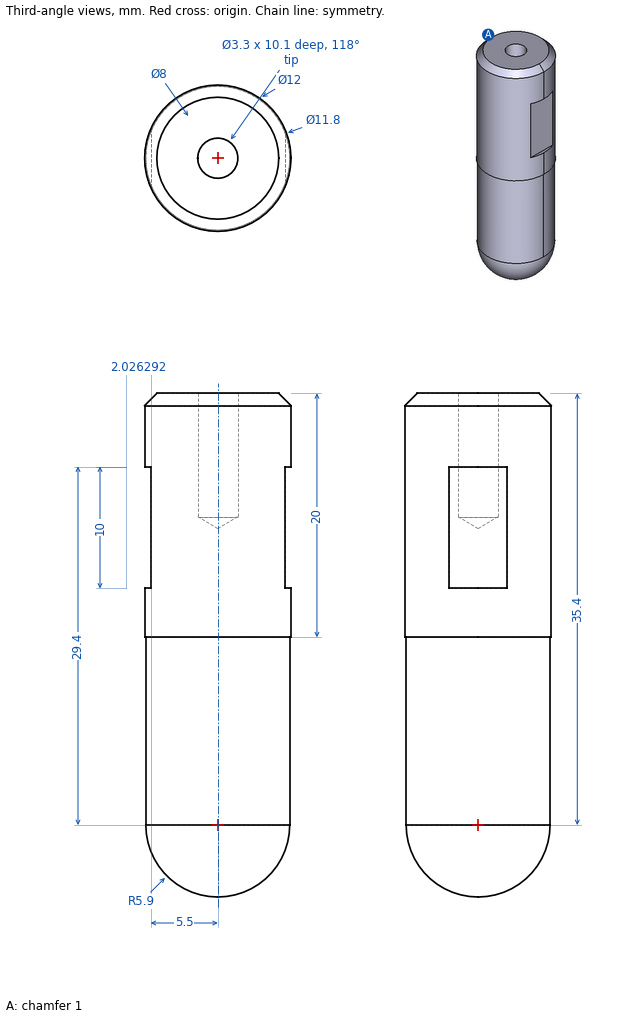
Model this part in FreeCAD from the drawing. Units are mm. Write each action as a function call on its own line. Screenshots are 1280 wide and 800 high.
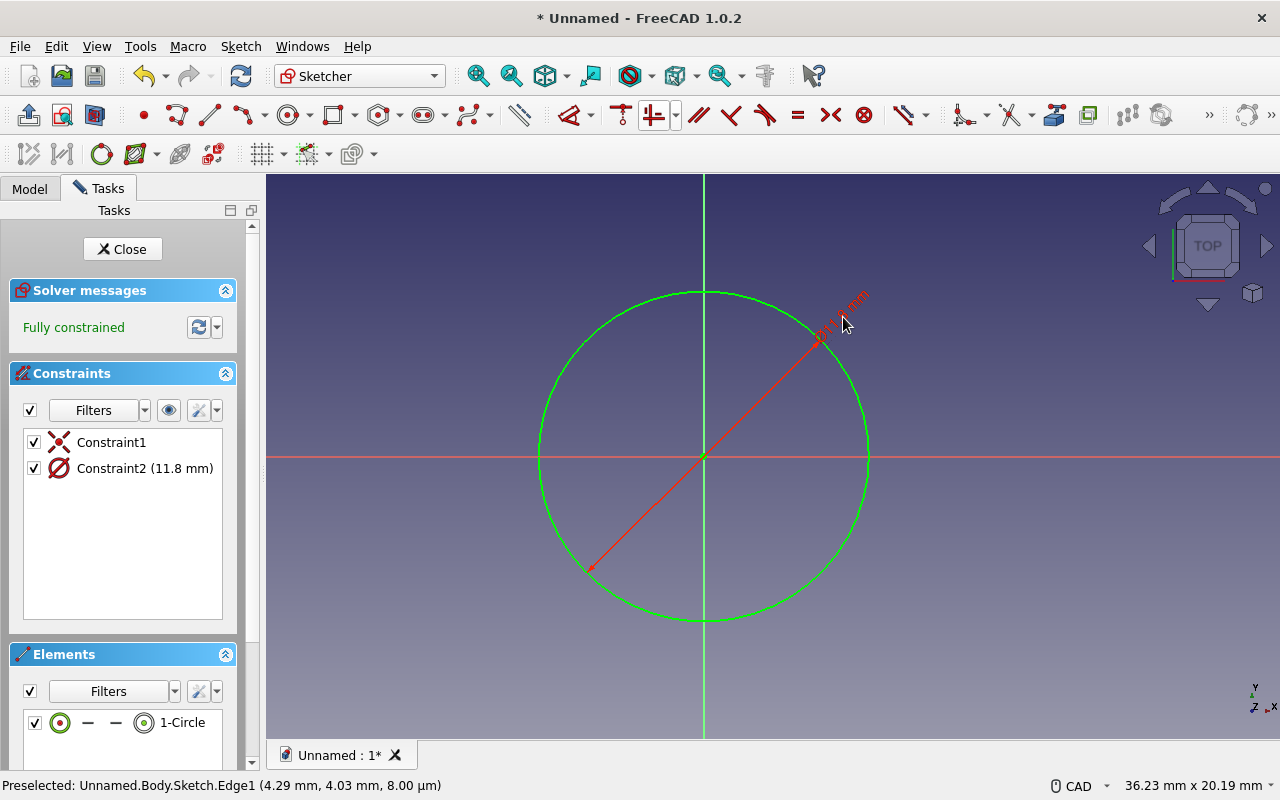
click(123, 249)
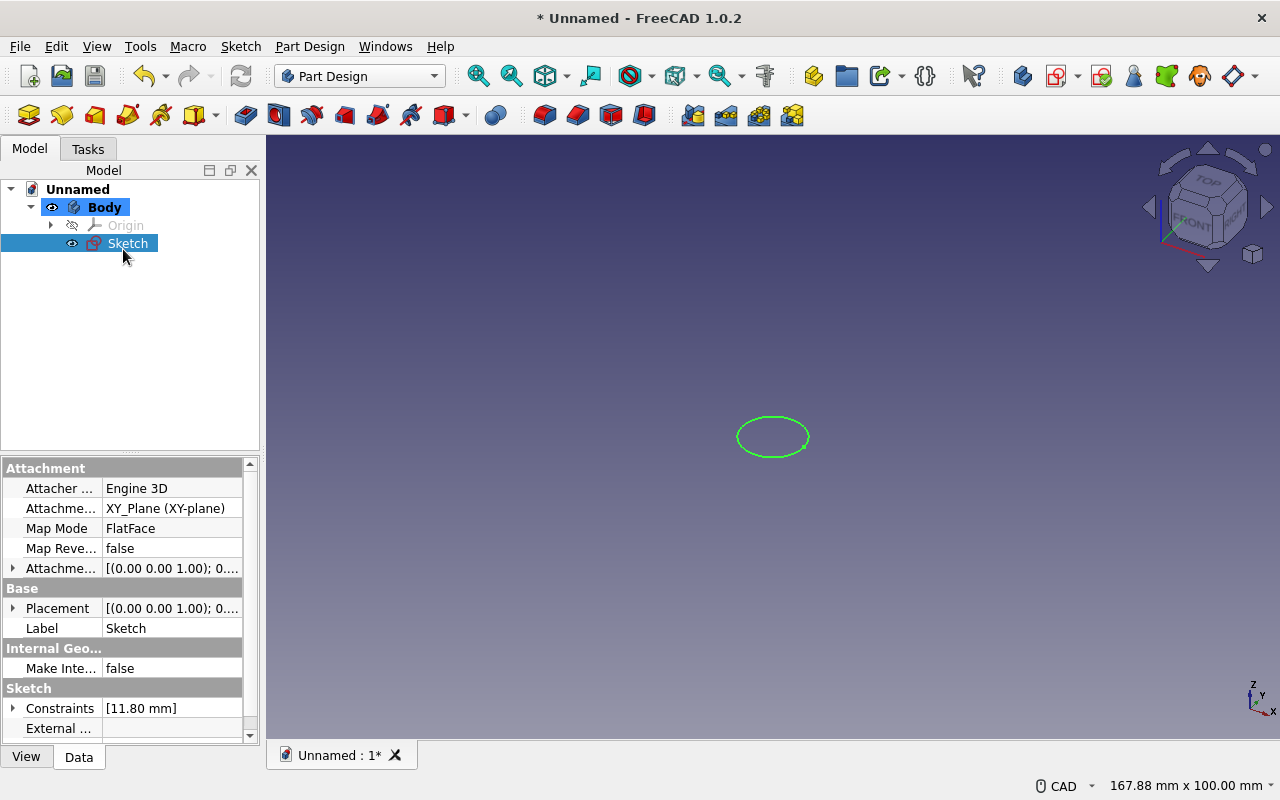
click(29, 116)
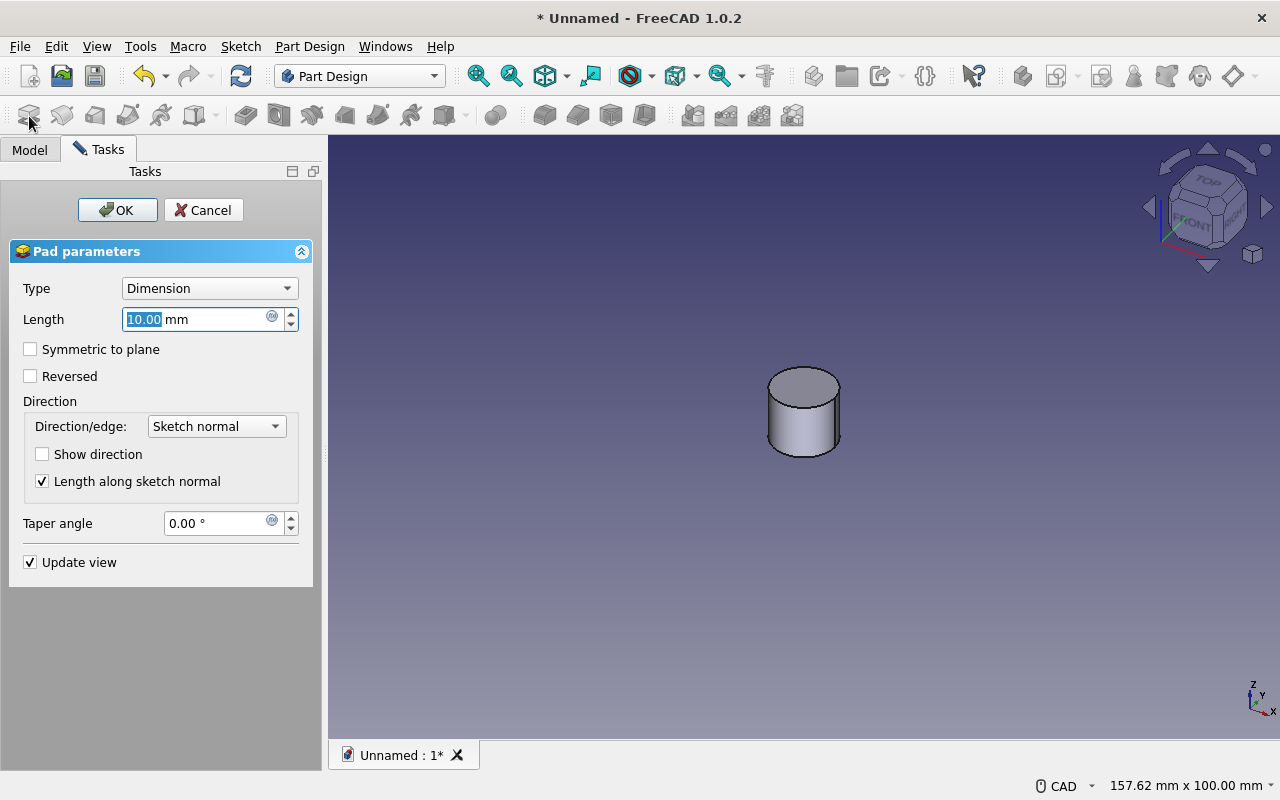
text(35.4)
key(Tab)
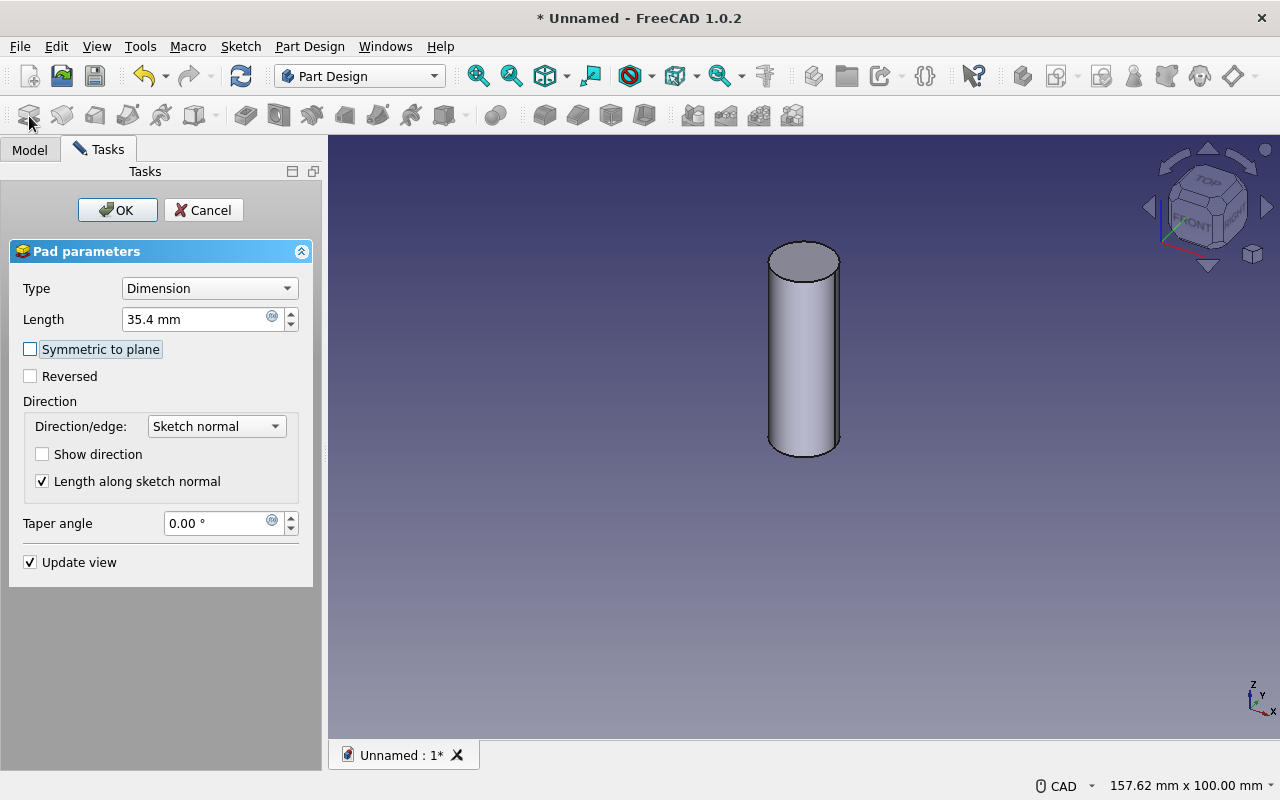
click(118, 210)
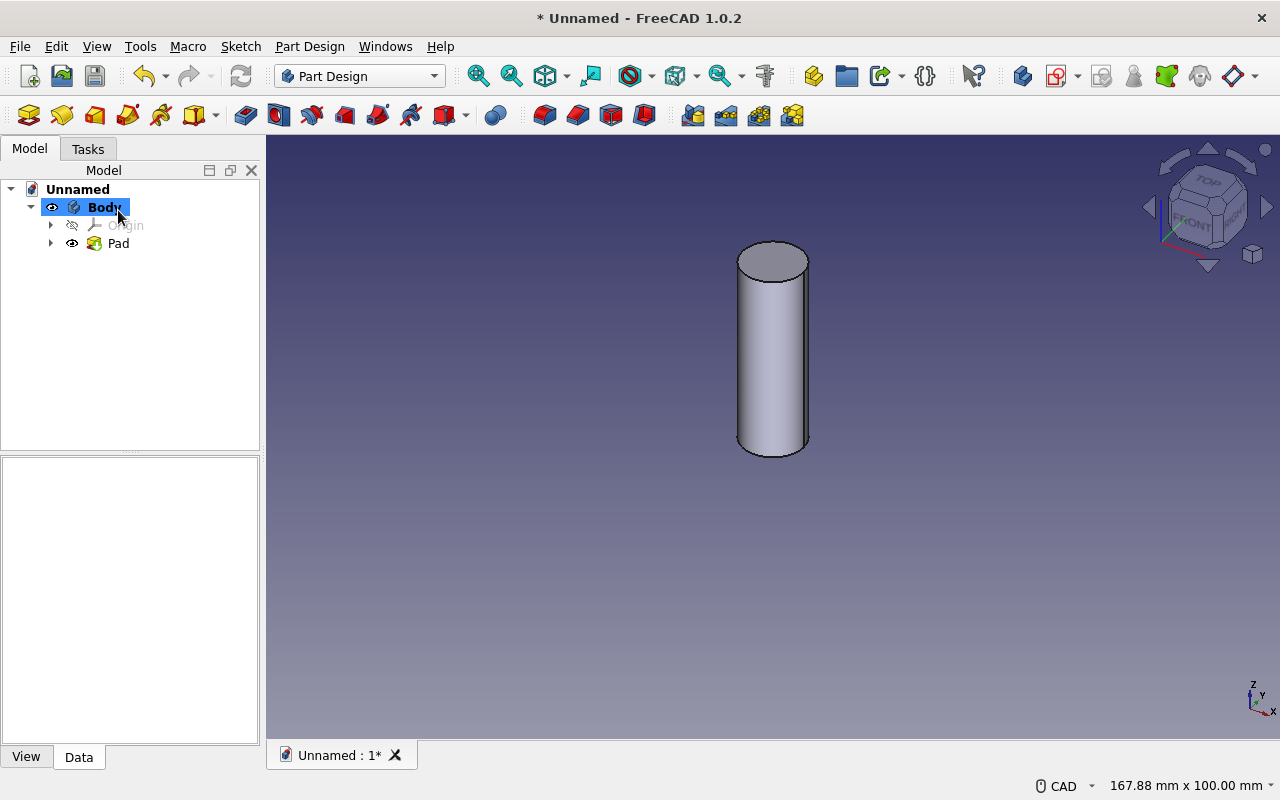
click(479, 76)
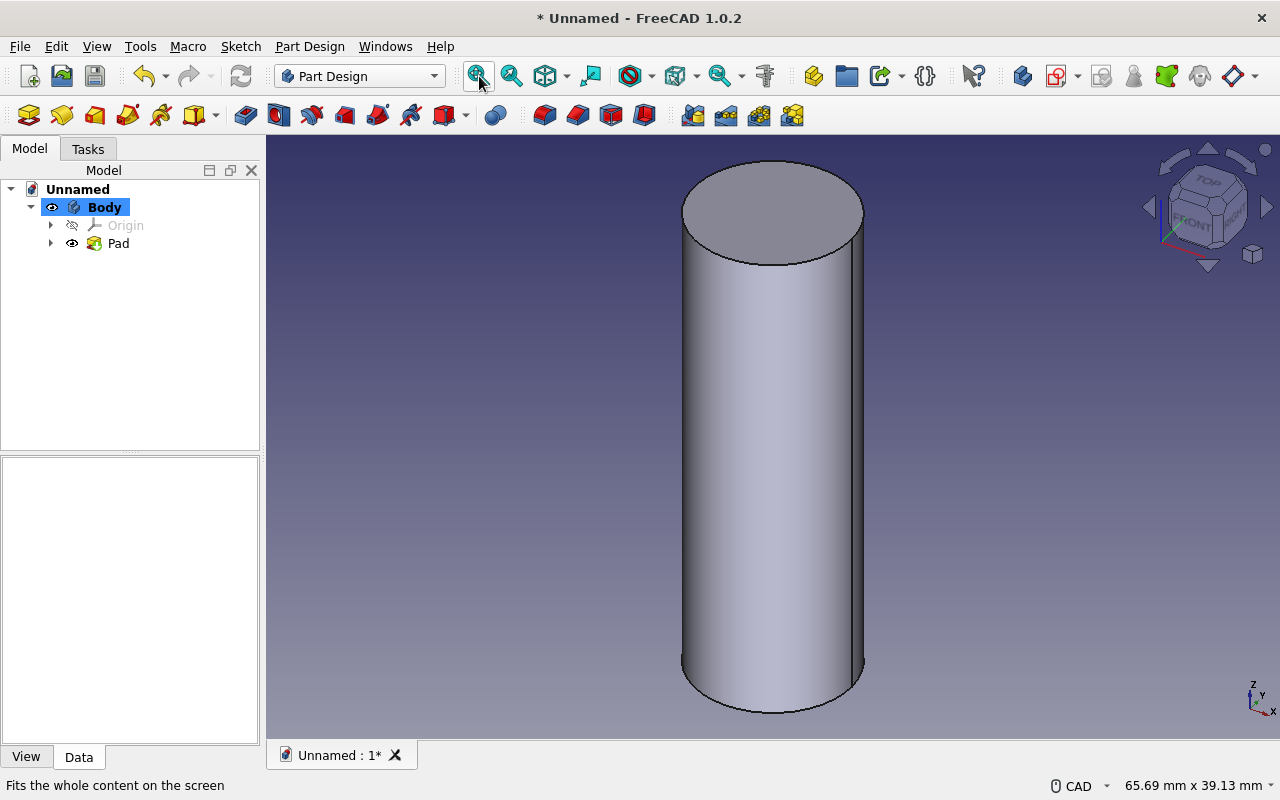
click(1056, 76)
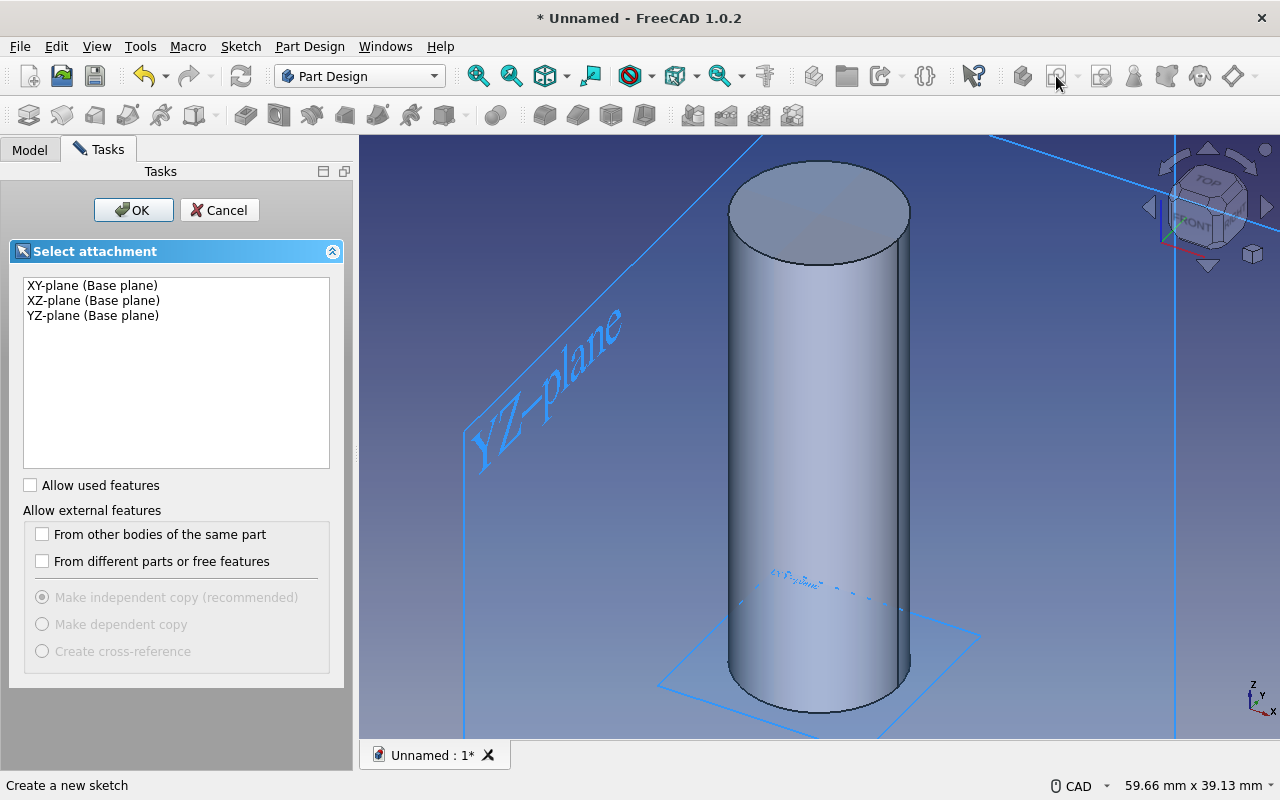
click(84, 300)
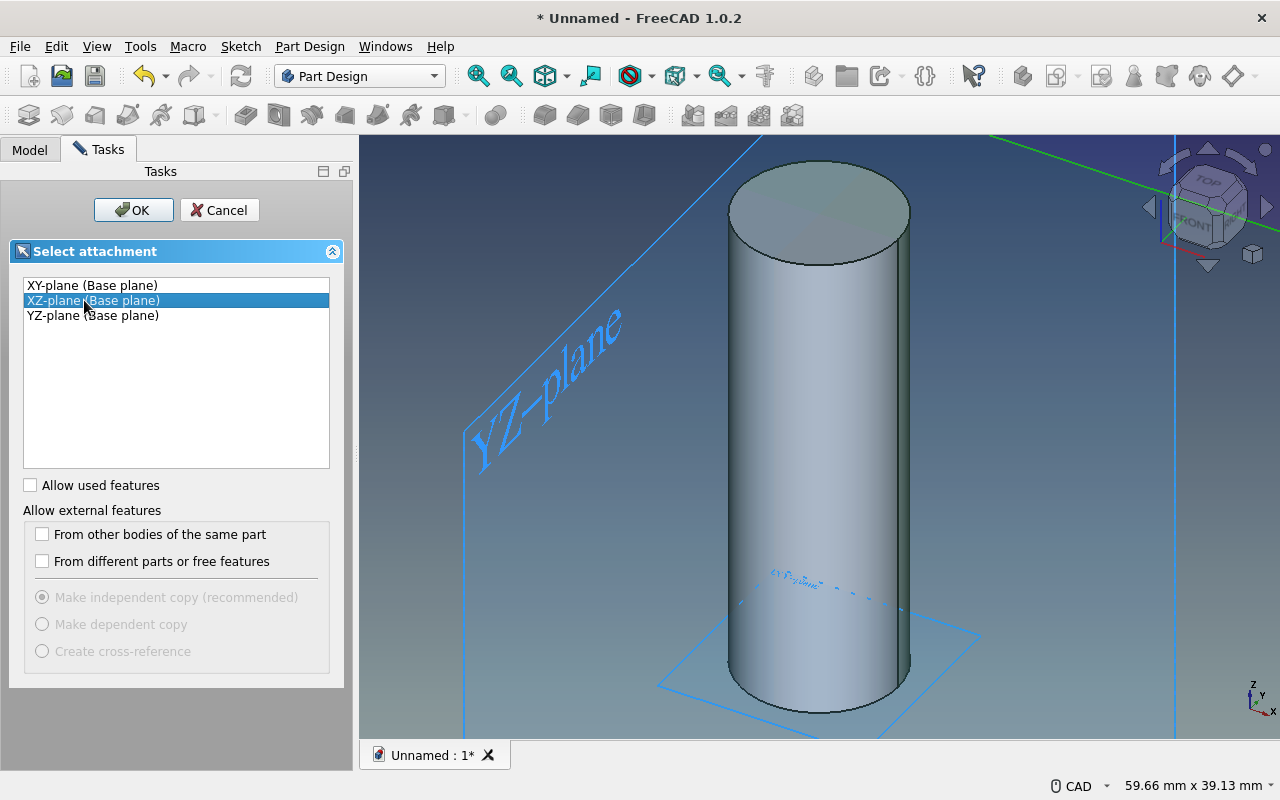
click(134, 210)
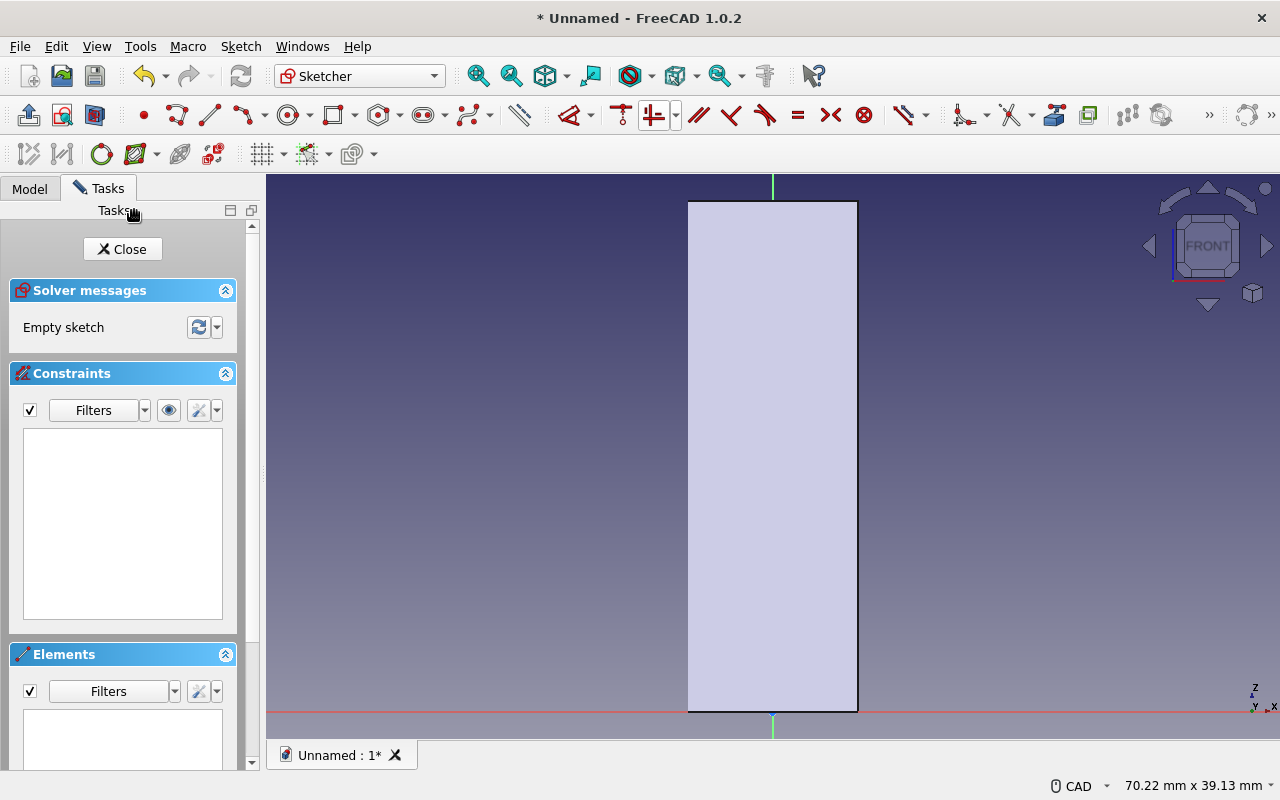
click(95, 116)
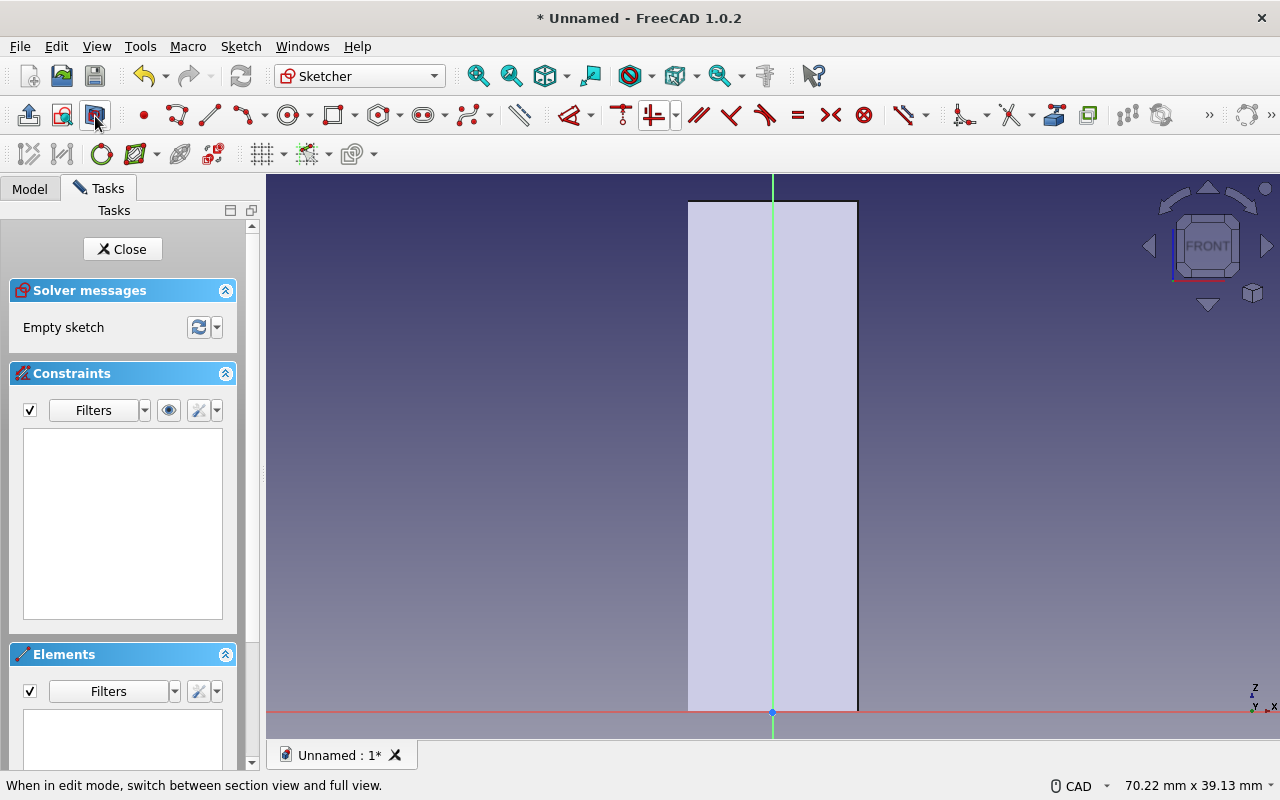
scroll(704, 456, down, 5)